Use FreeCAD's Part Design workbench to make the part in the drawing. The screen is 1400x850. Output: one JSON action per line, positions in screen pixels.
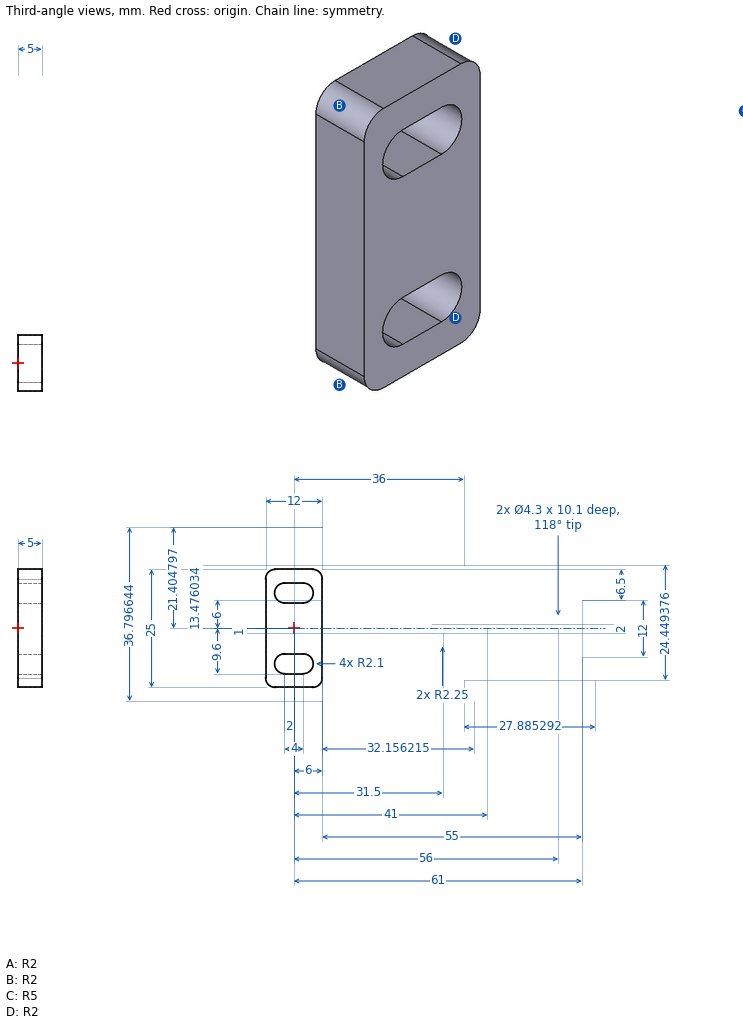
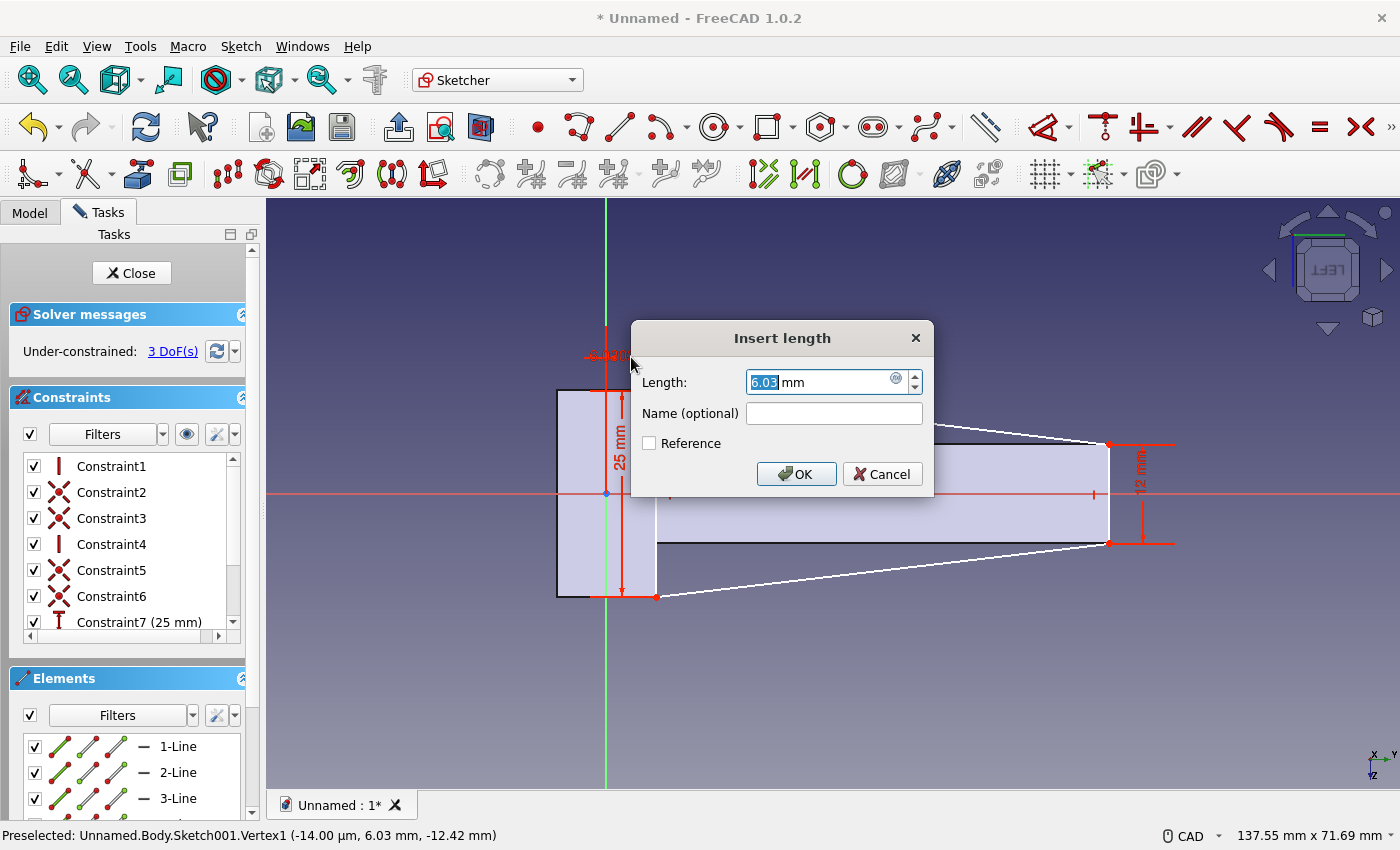
{"action": "type", "text": "6"}
{"action": "key", "text": "Return"}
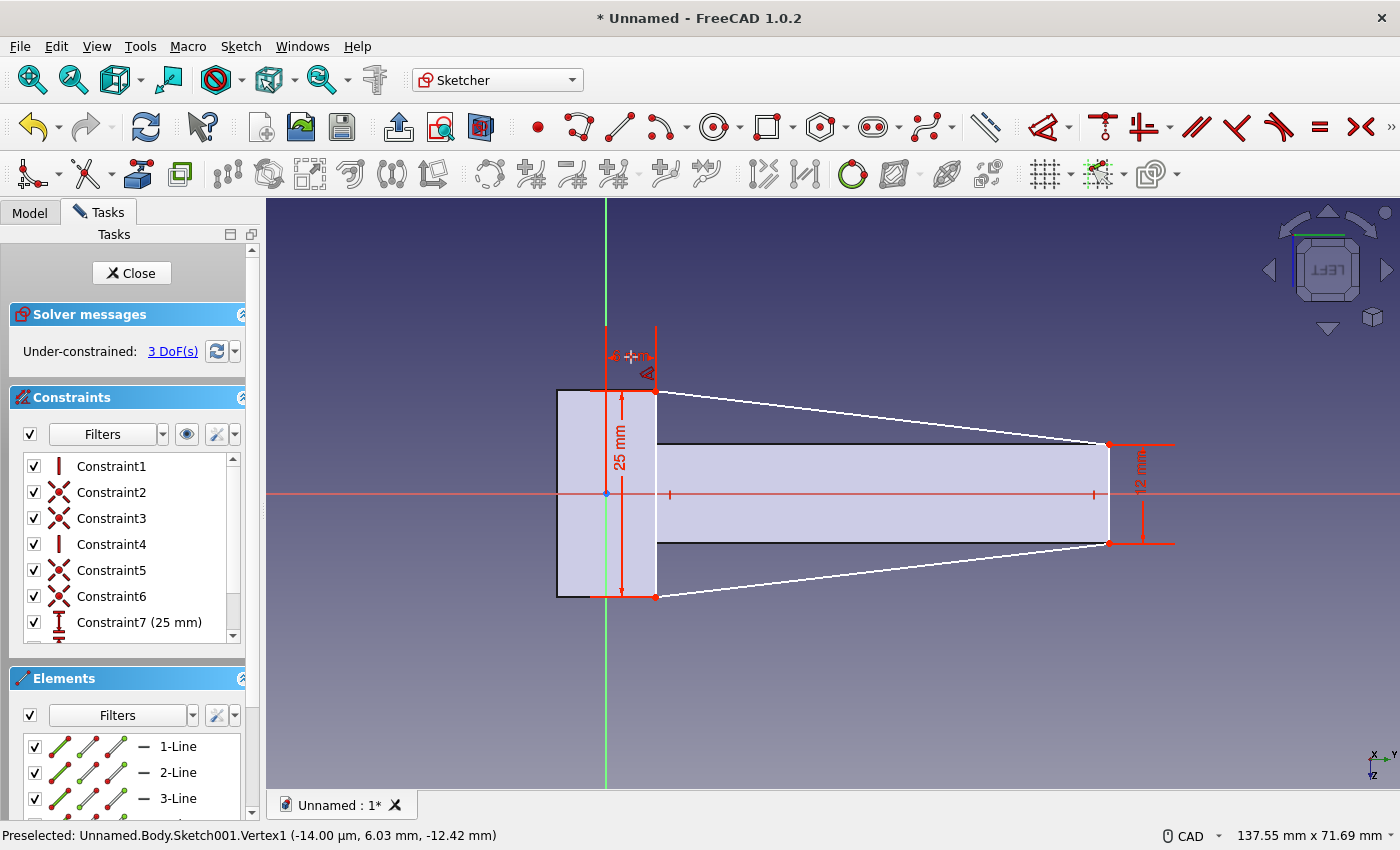
{"action": "left_click", "coordinate": [1109, 544]}
{"action": "left_click", "coordinate": [572, 519]}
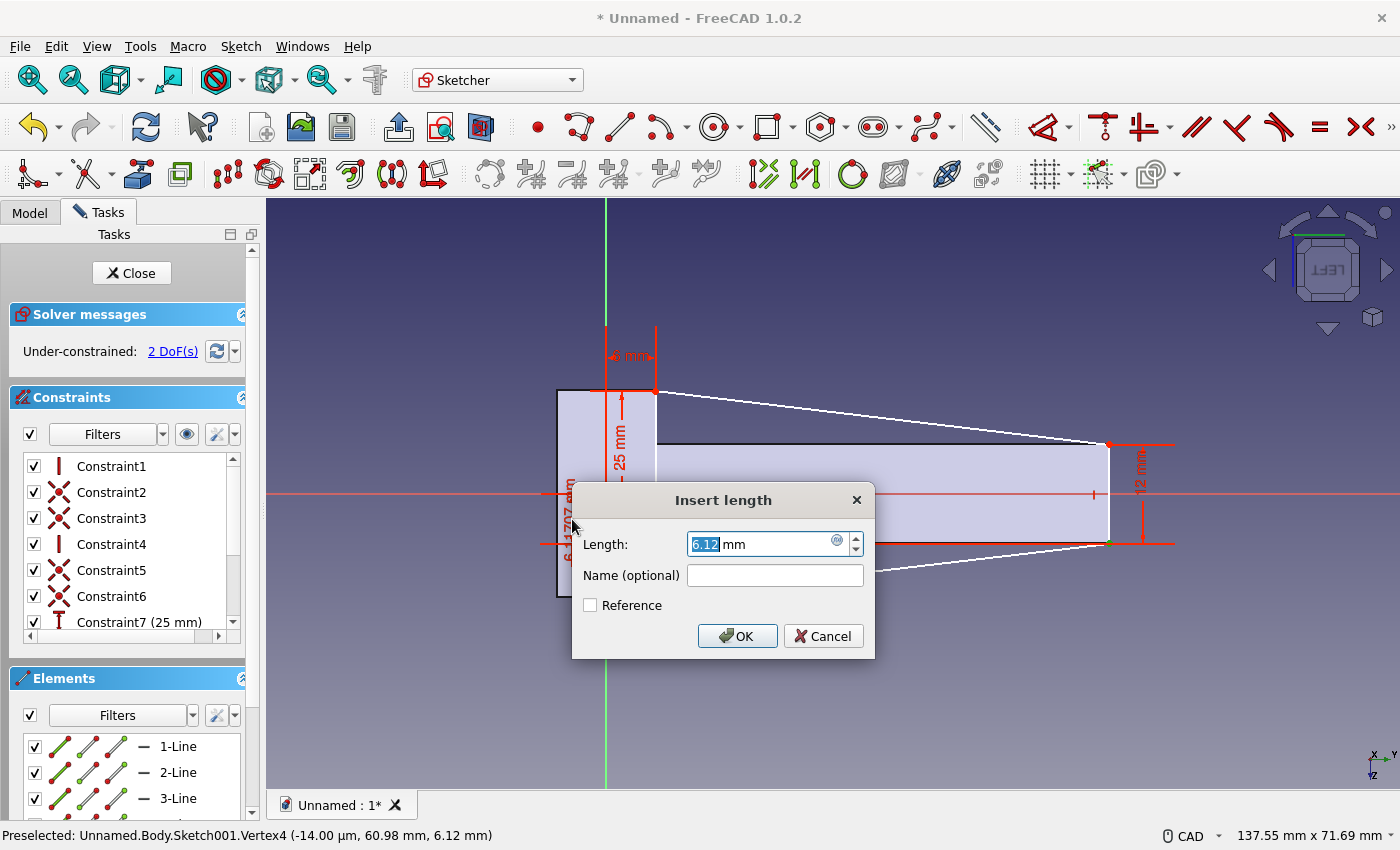
{"action": "type", "text": "6"}
{"action": "key", "text": "Return"}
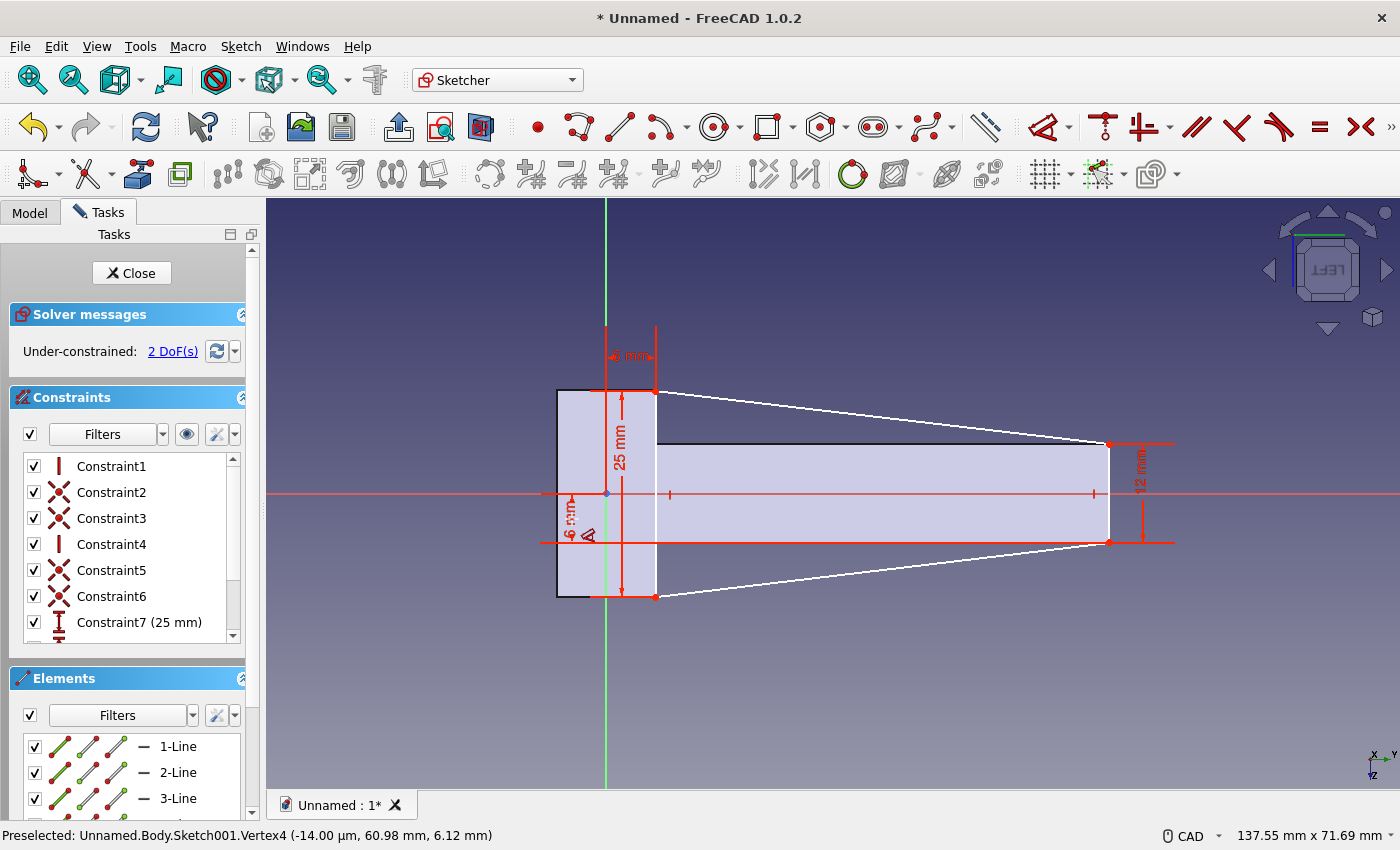
{"action": "left_click", "coordinate": [1109, 543]}
{"action": "left_click", "coordinate": [973, 577]}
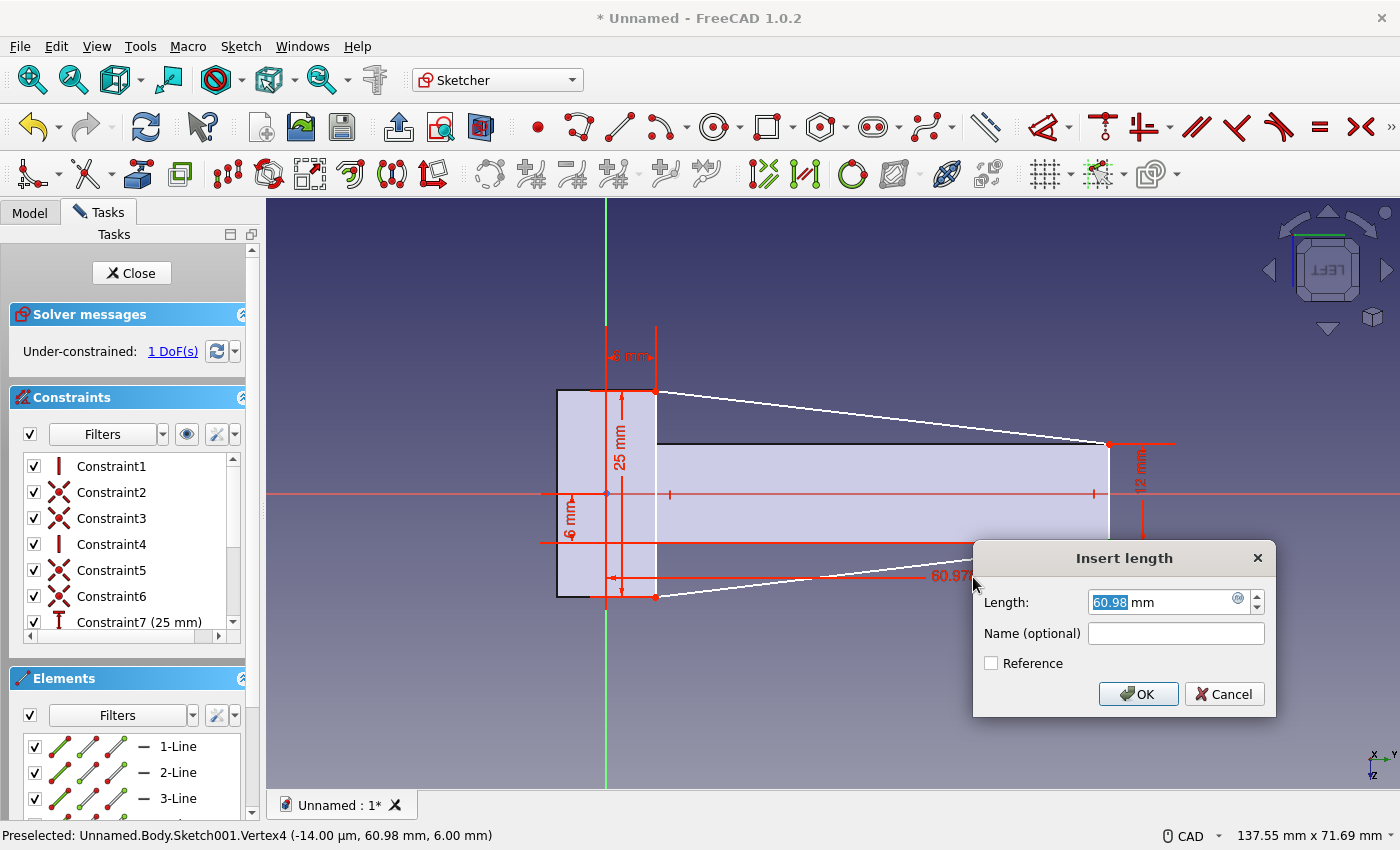
{"action": "type", "text": "61"}
{"action": "key", "text": "Return"}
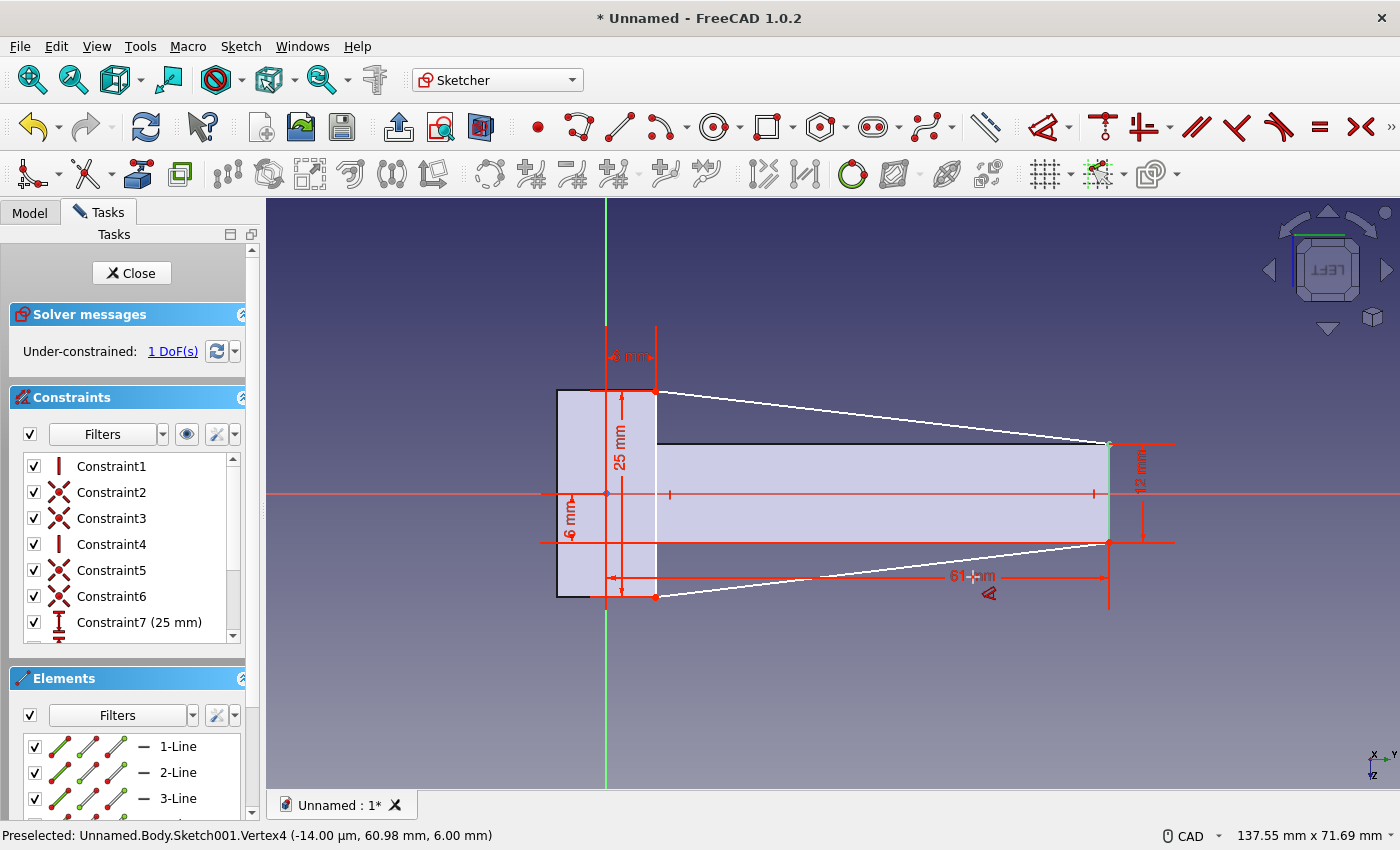
{"action": "left_click", "coordinate": [792, 581]}
{"action": "left_click", "coordinate": [1143, 570]}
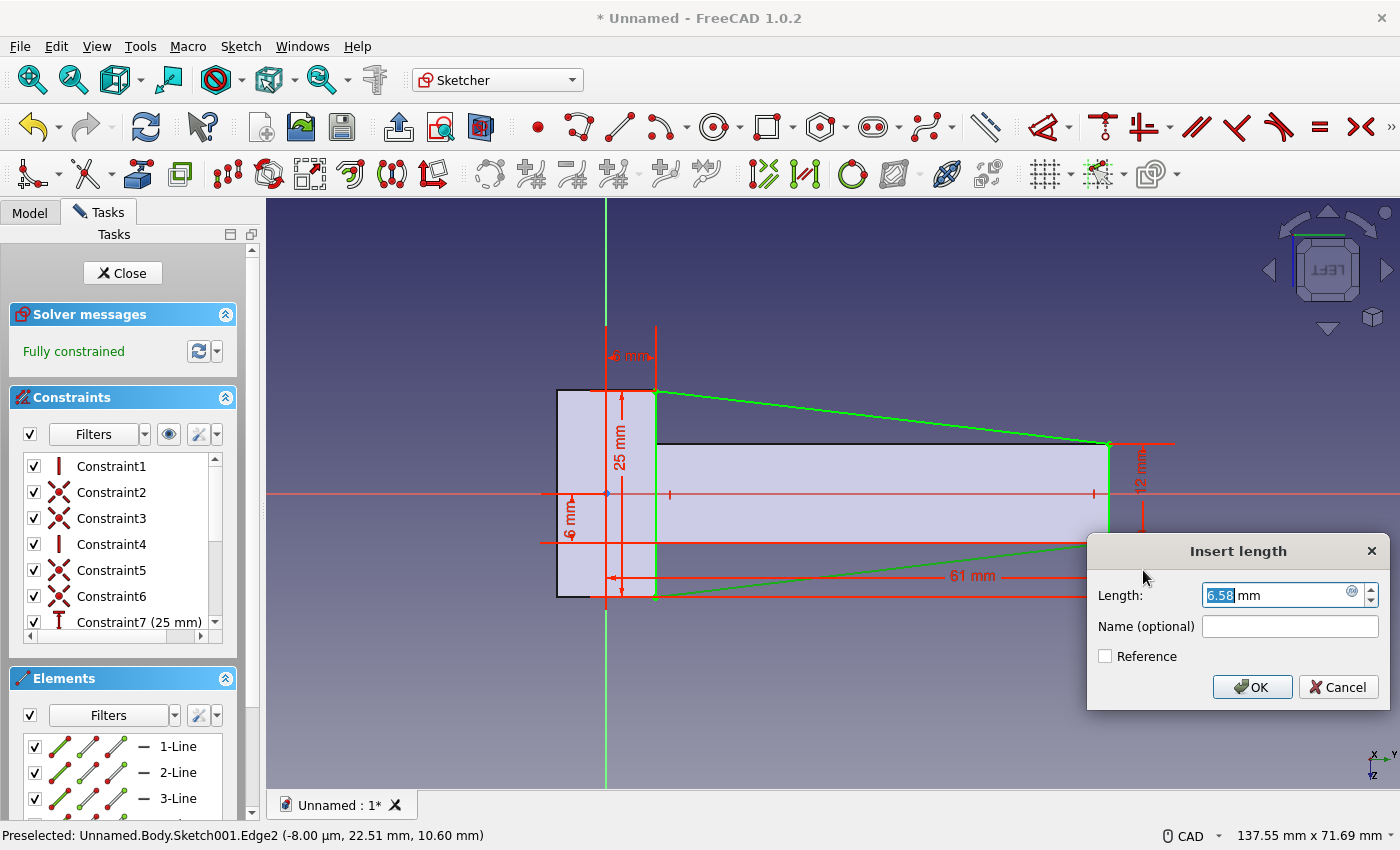
{"action": "type", "text": "6.5"}
{"action": "key", "text": "Return"}
{"action": "key", "text": "Escape"}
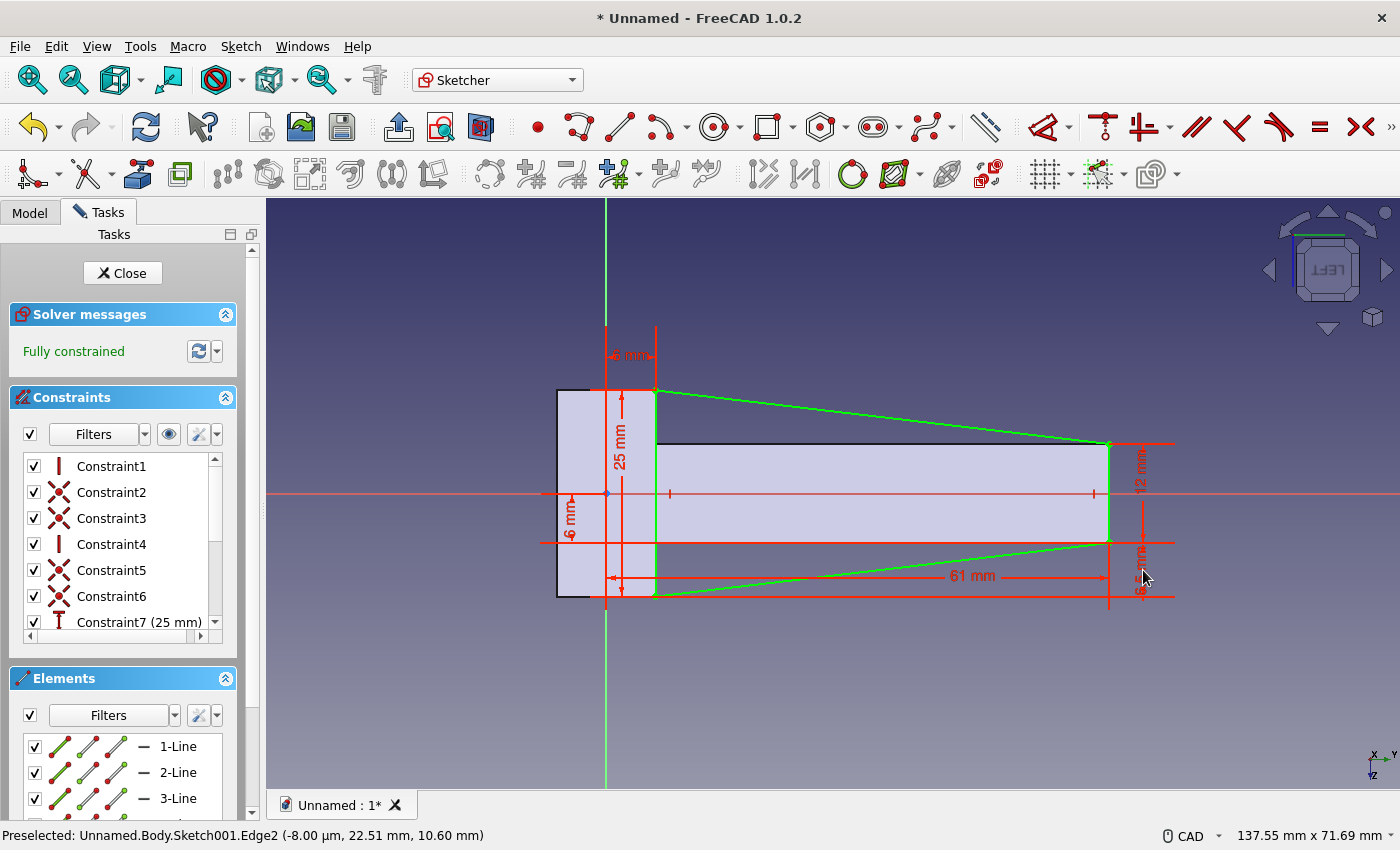
{"action": "left_click", "coordinate": [123, 273]}